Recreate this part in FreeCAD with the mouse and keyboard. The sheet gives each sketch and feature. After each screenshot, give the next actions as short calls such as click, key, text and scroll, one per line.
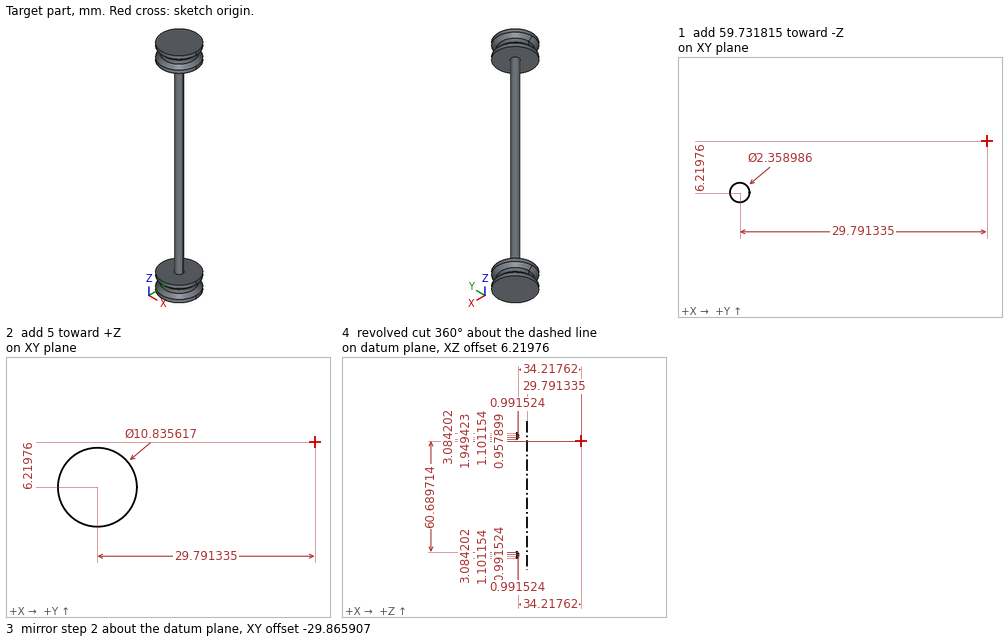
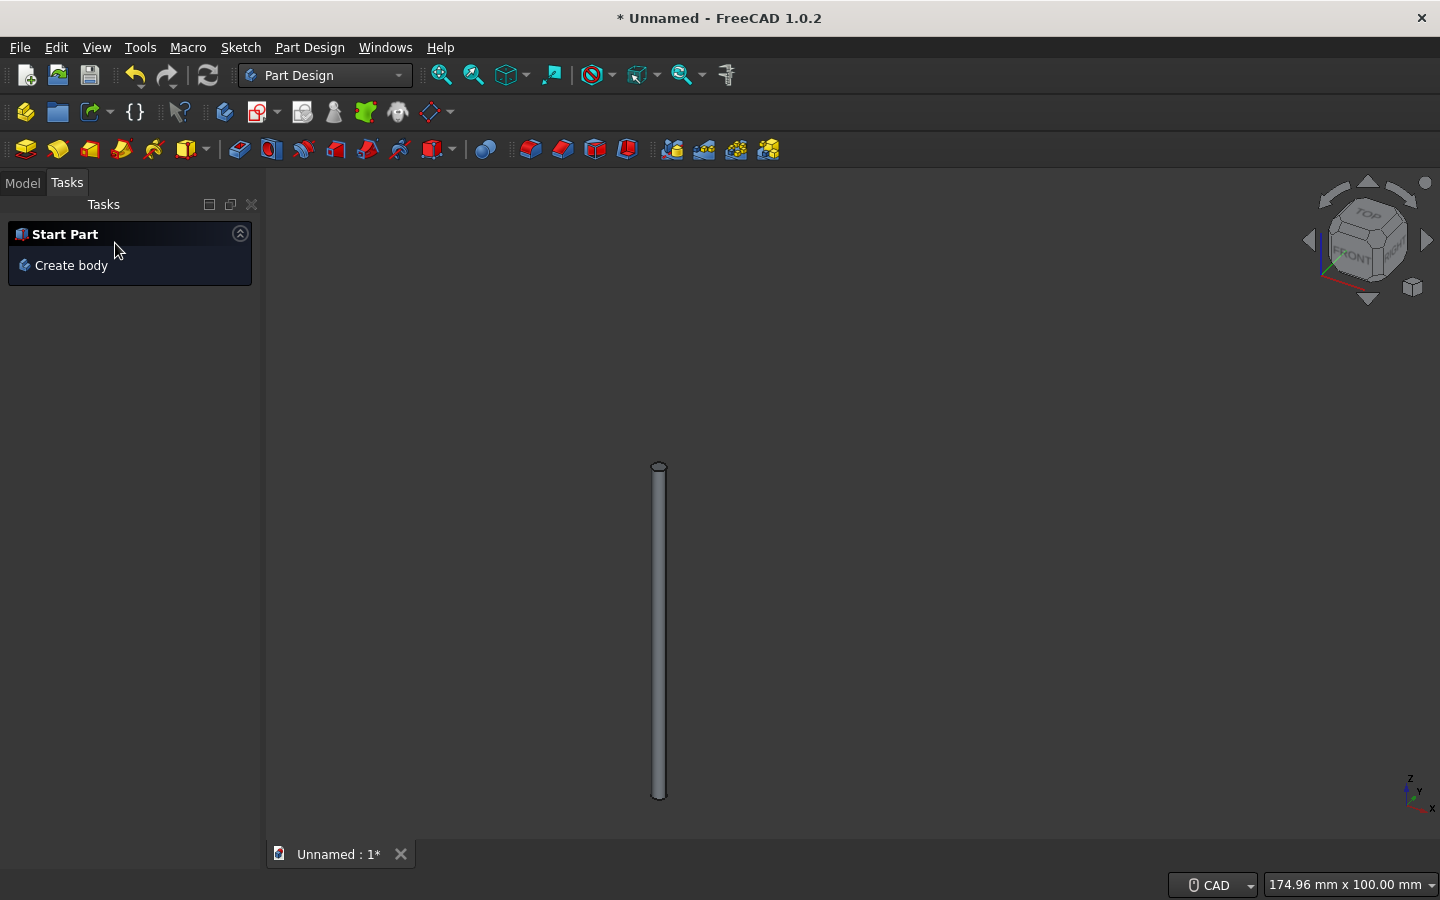
click(258, 112)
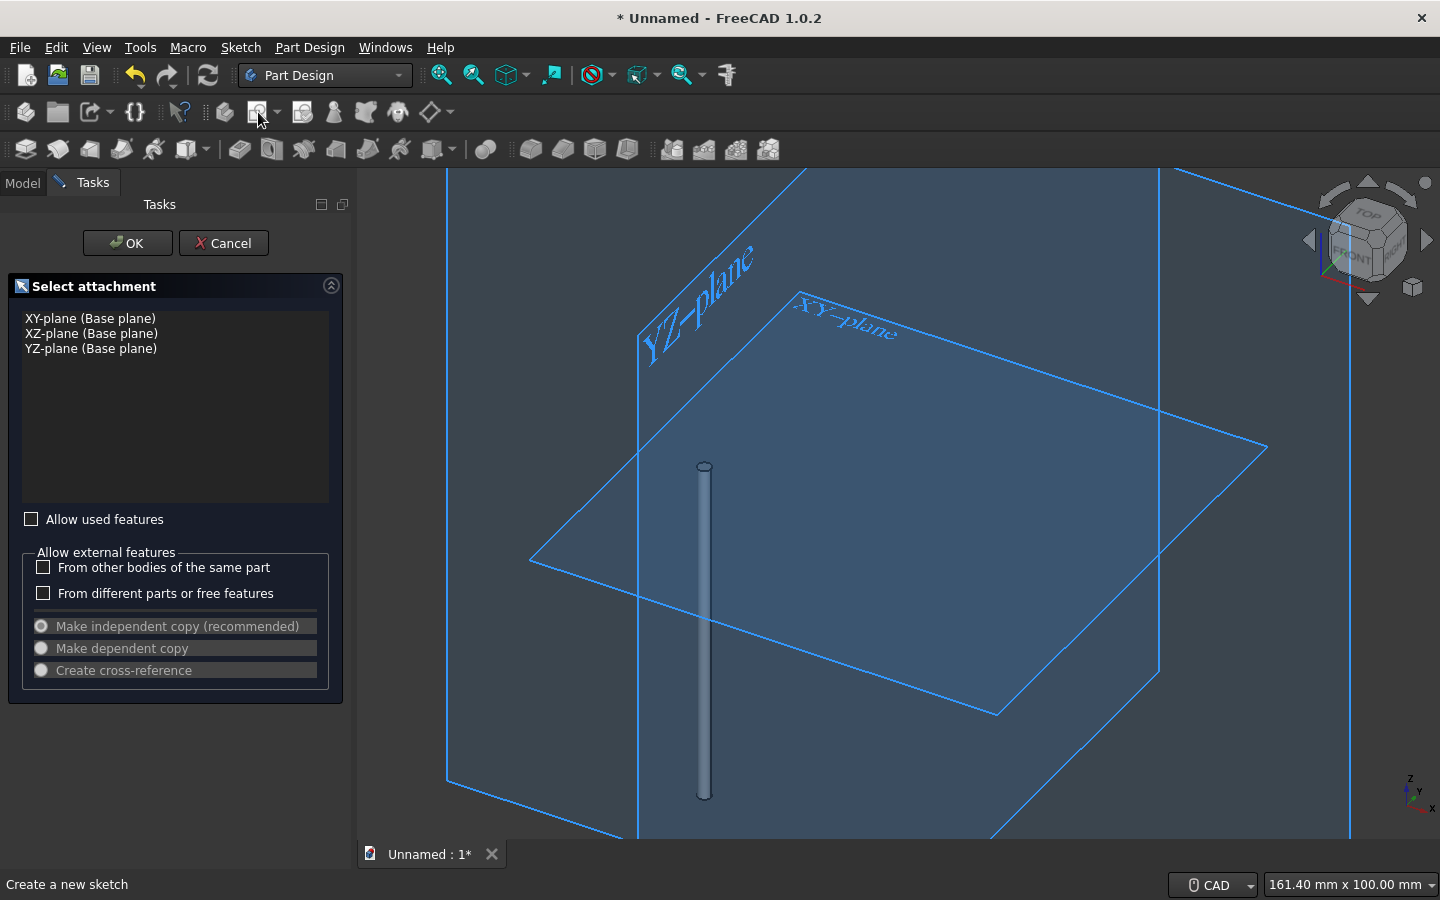
click(82, 318)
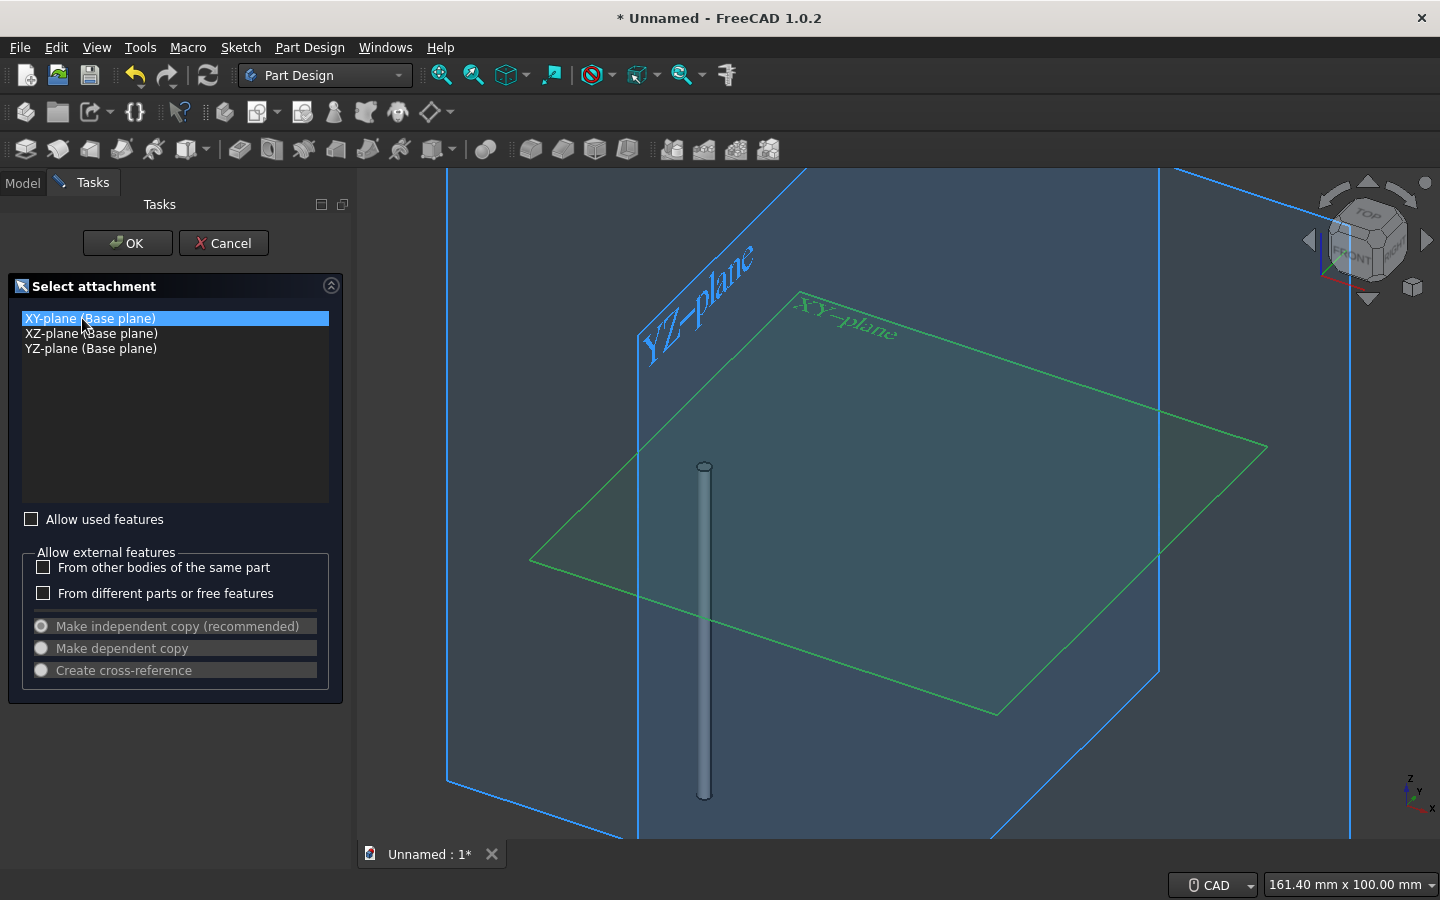
click(128, 243)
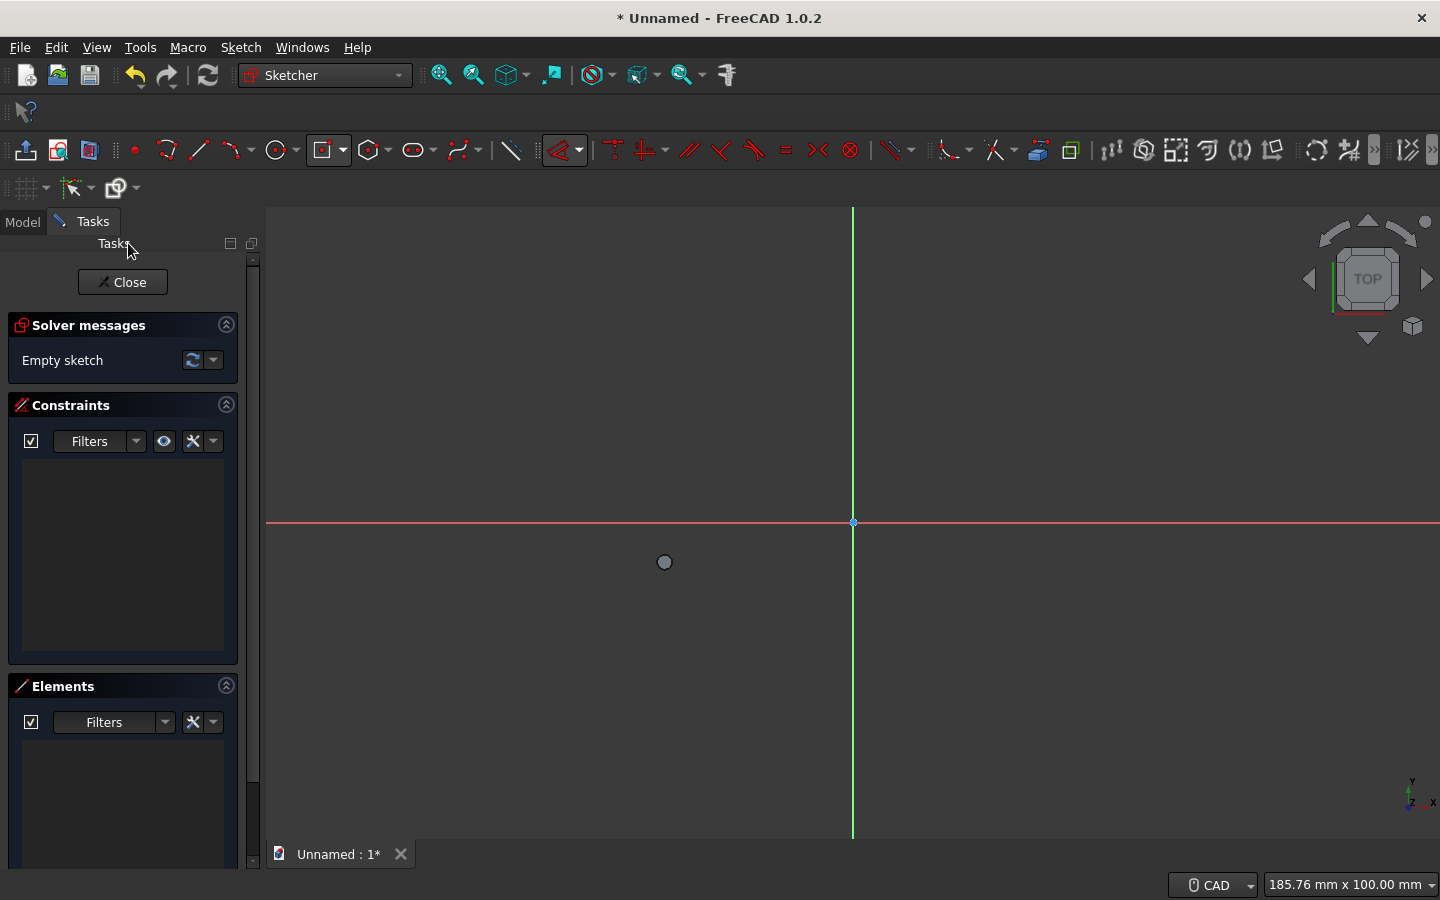
scroll(641, 570, up, 9)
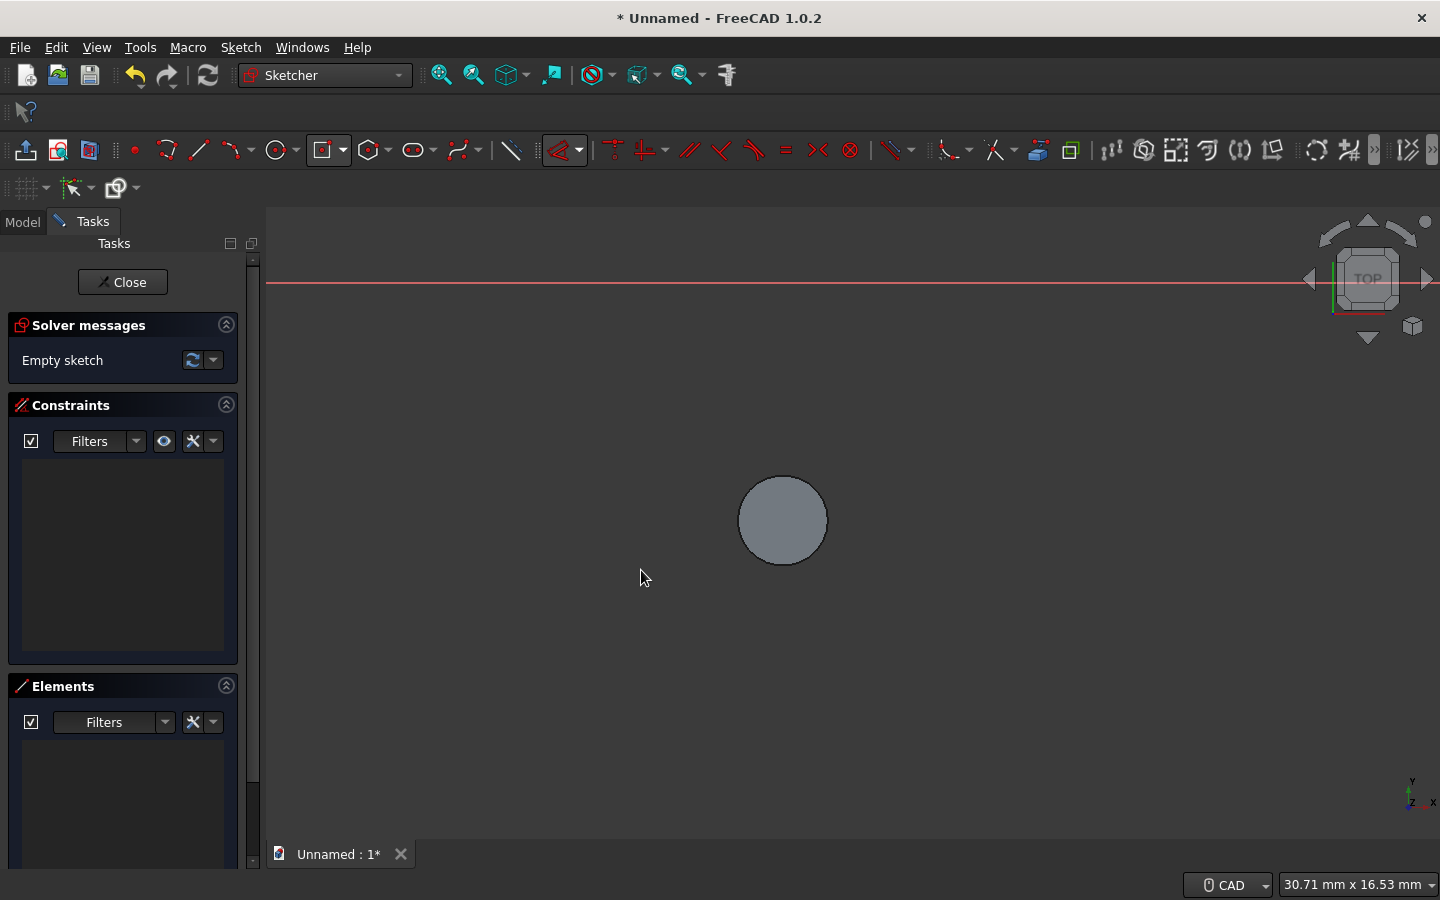
key(g)
key(c)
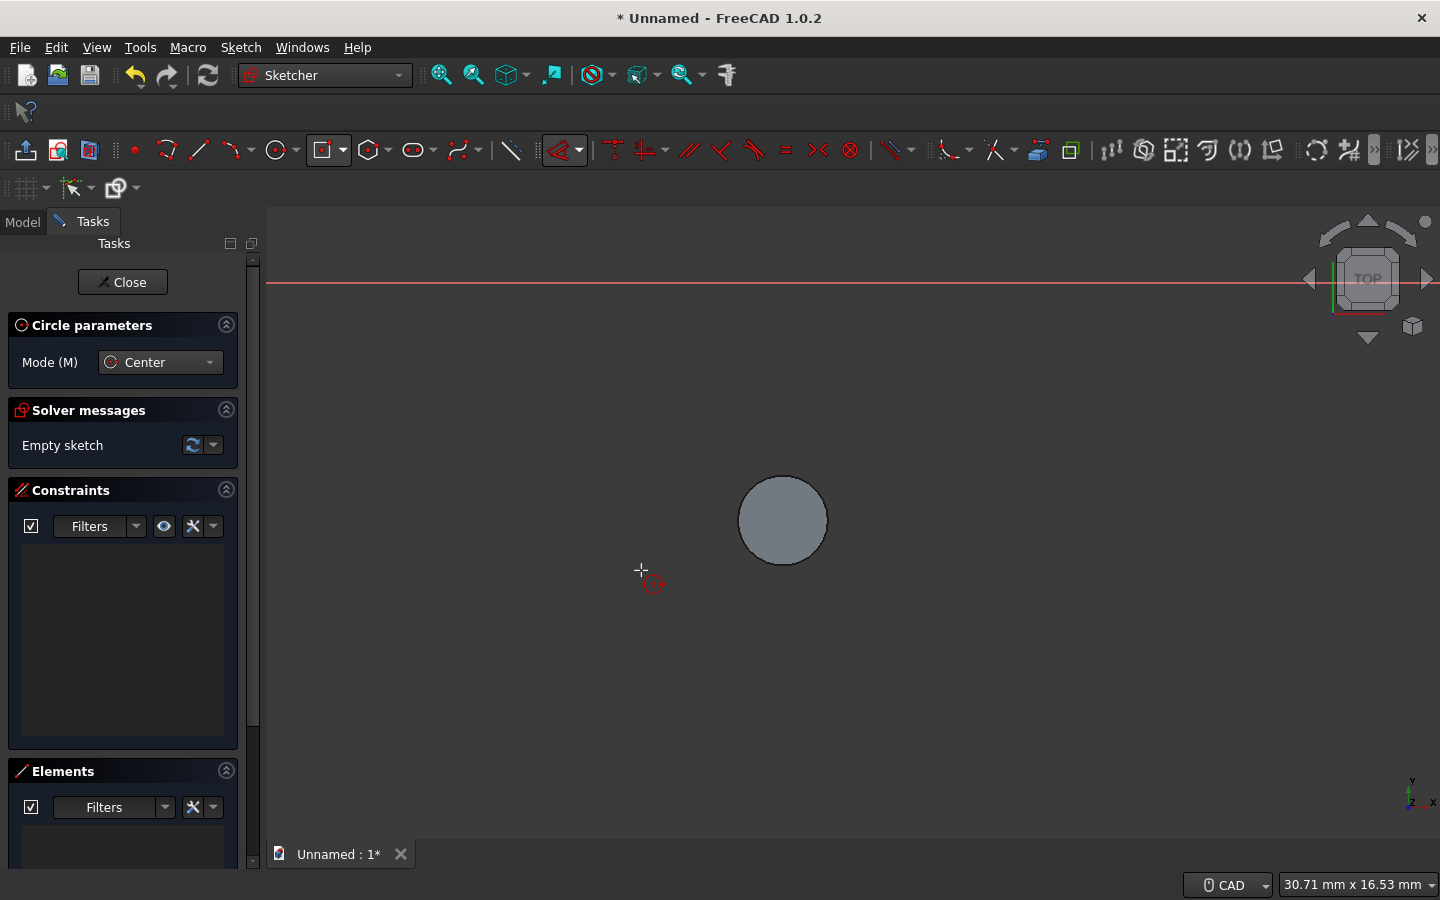
click(783, 521)
click(929, 374)
key(Escape)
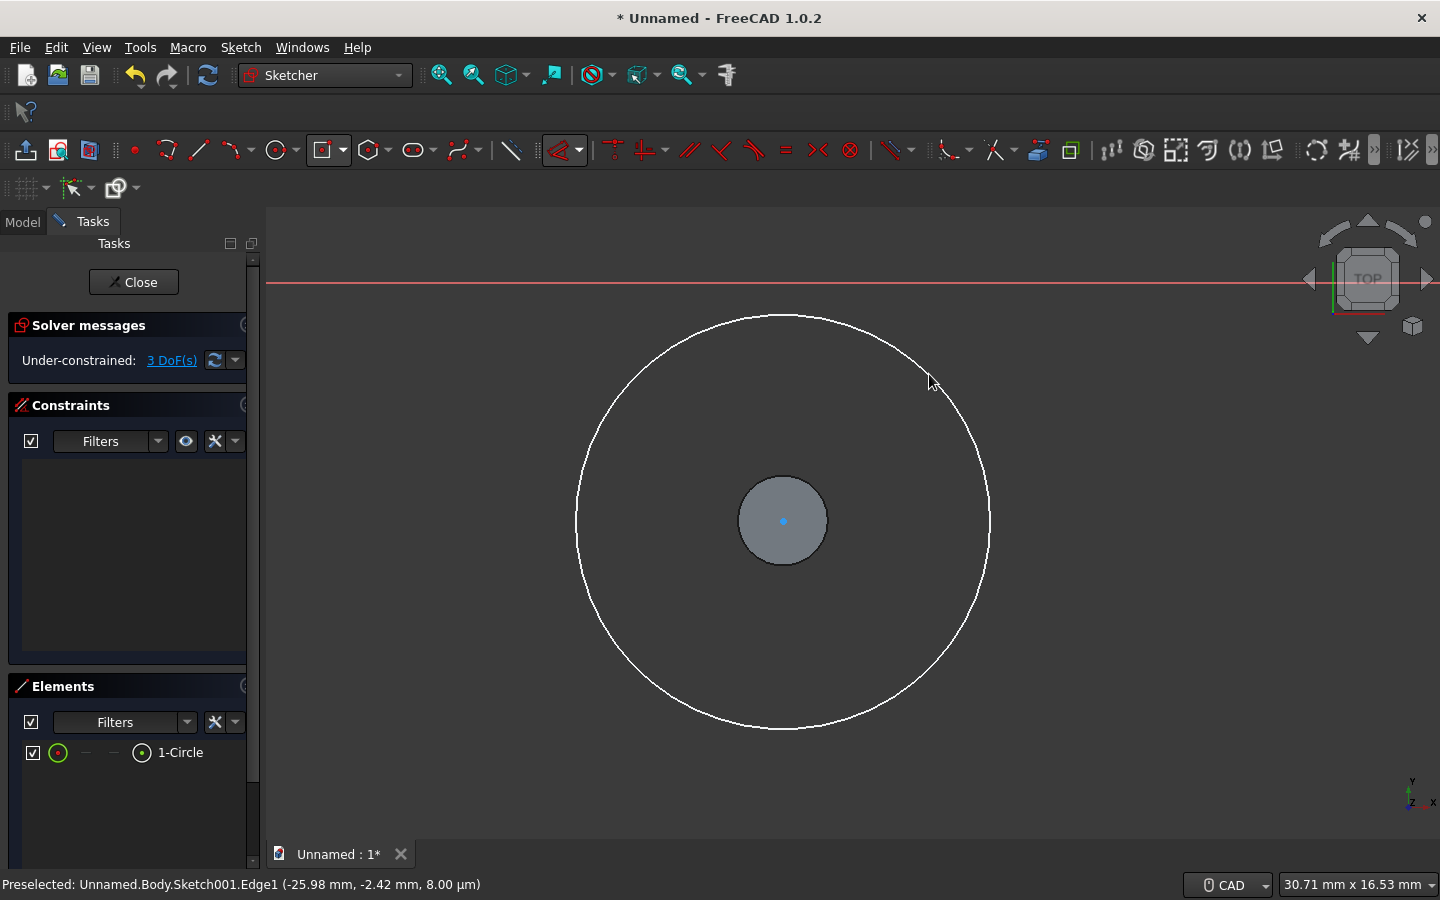
click(929, 375)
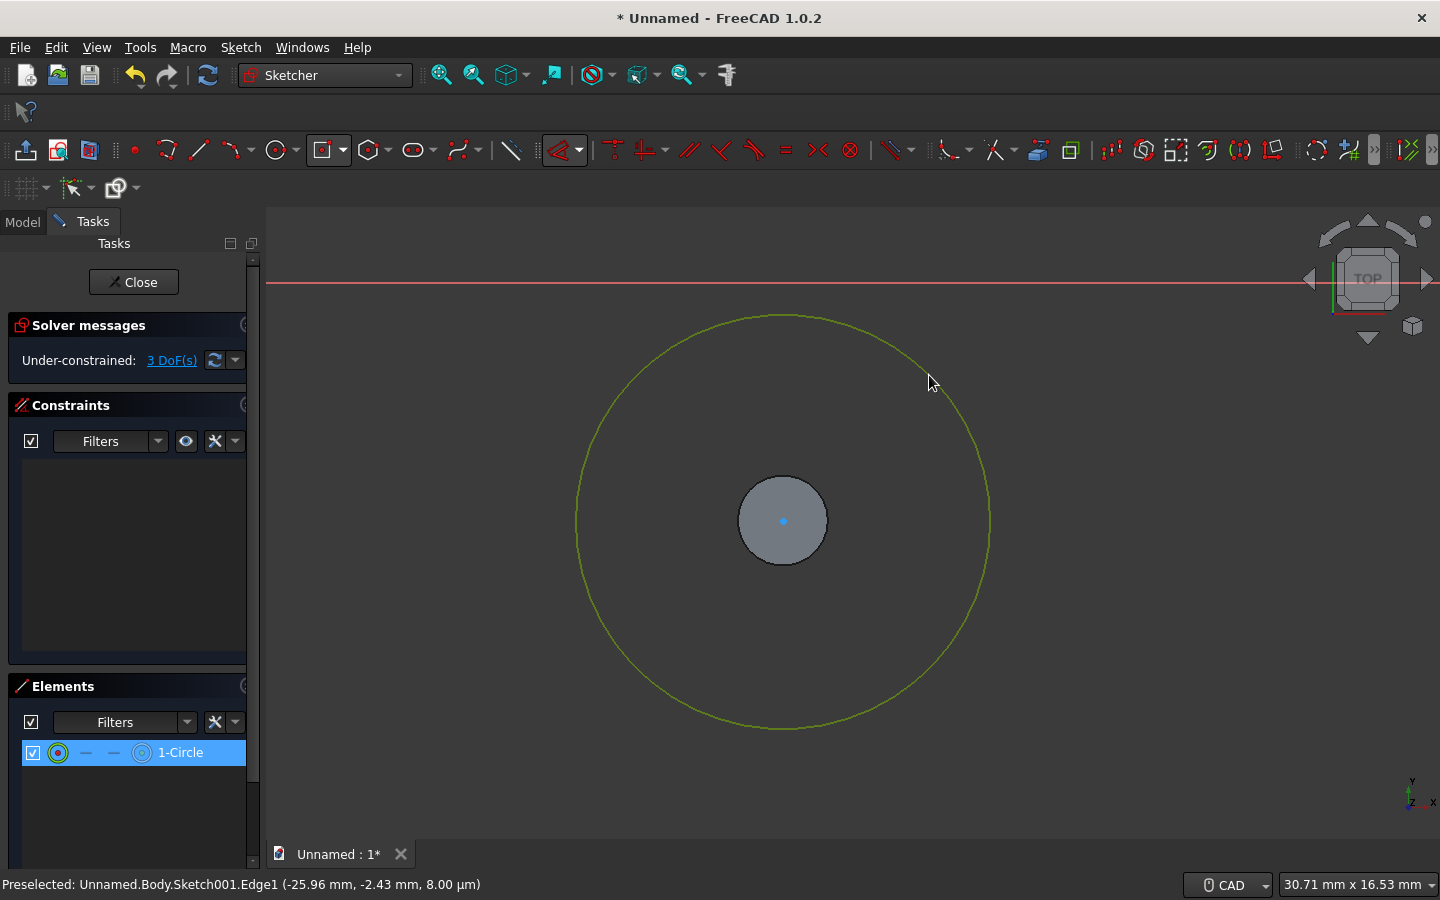
key(k)
key(o)